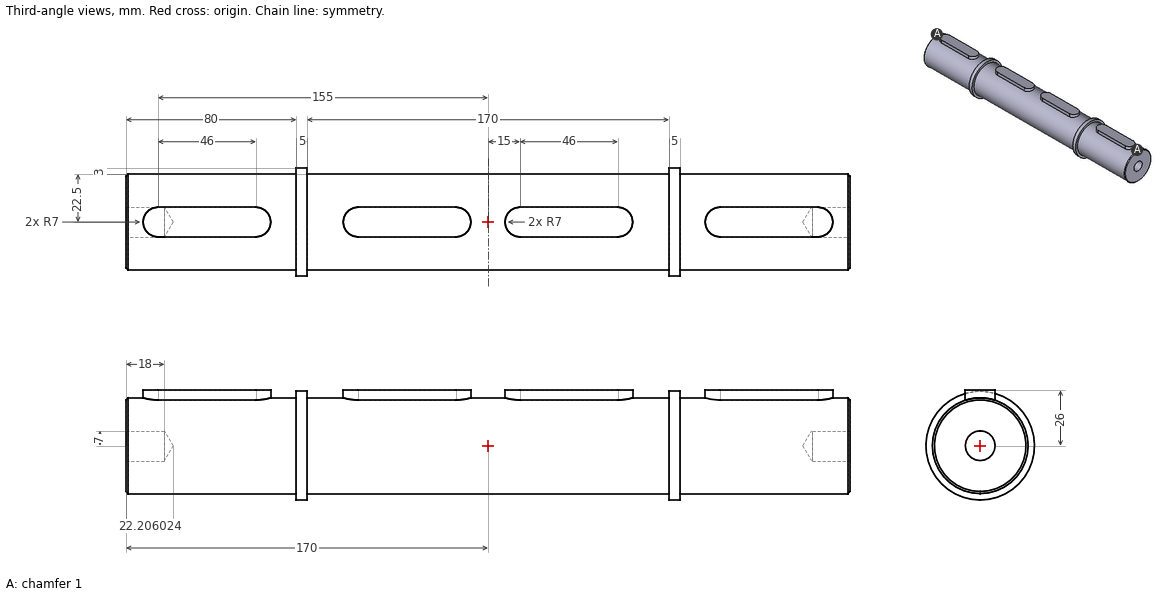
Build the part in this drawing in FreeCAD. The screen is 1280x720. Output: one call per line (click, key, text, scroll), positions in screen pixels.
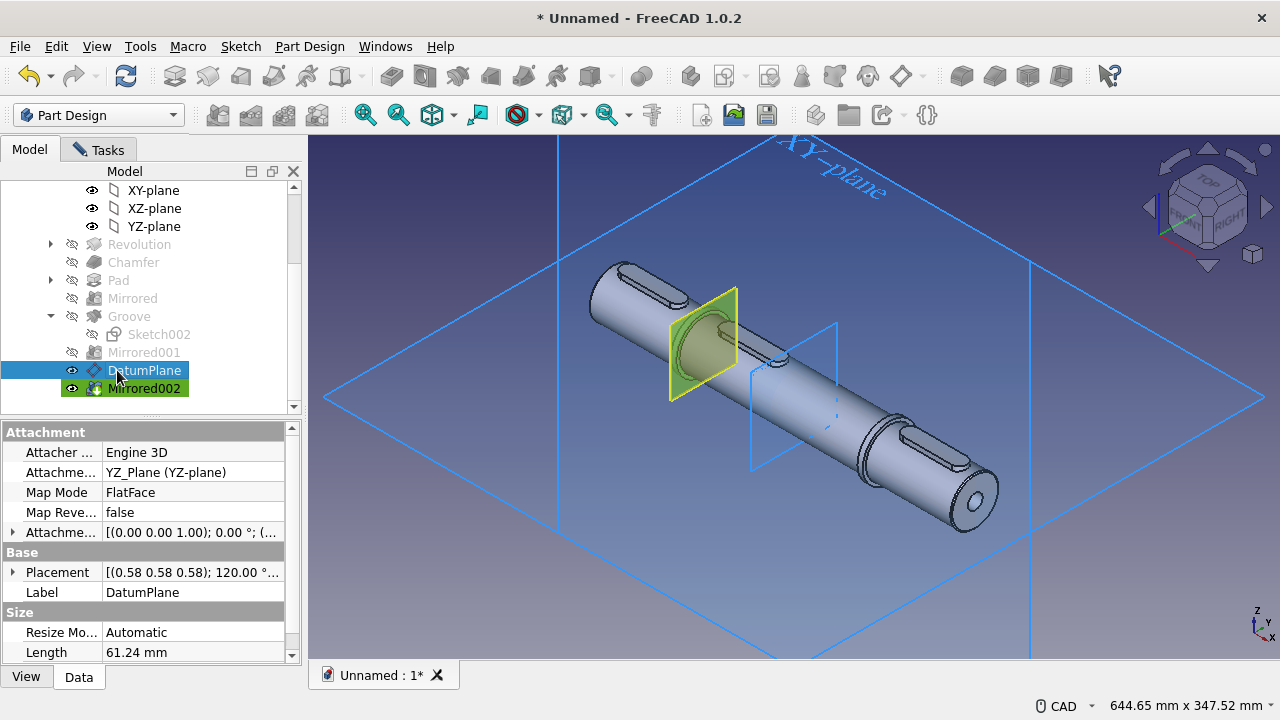
click(98, 149)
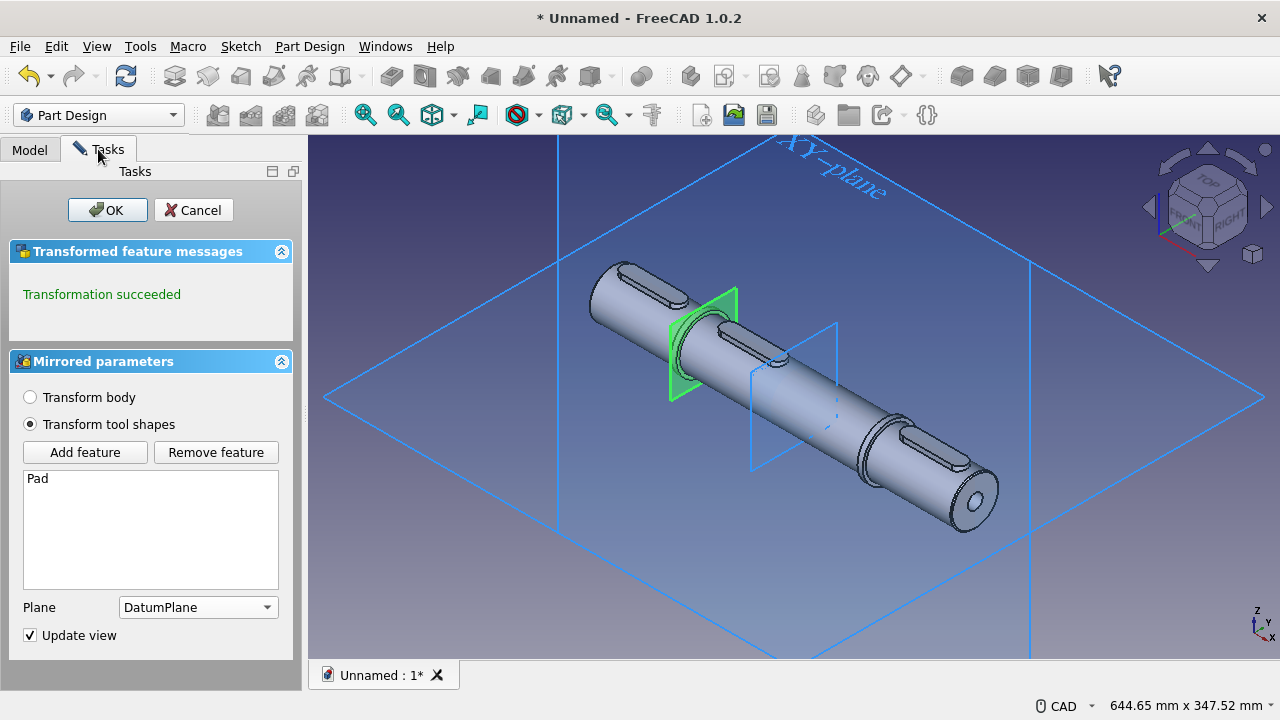
click(108, 210)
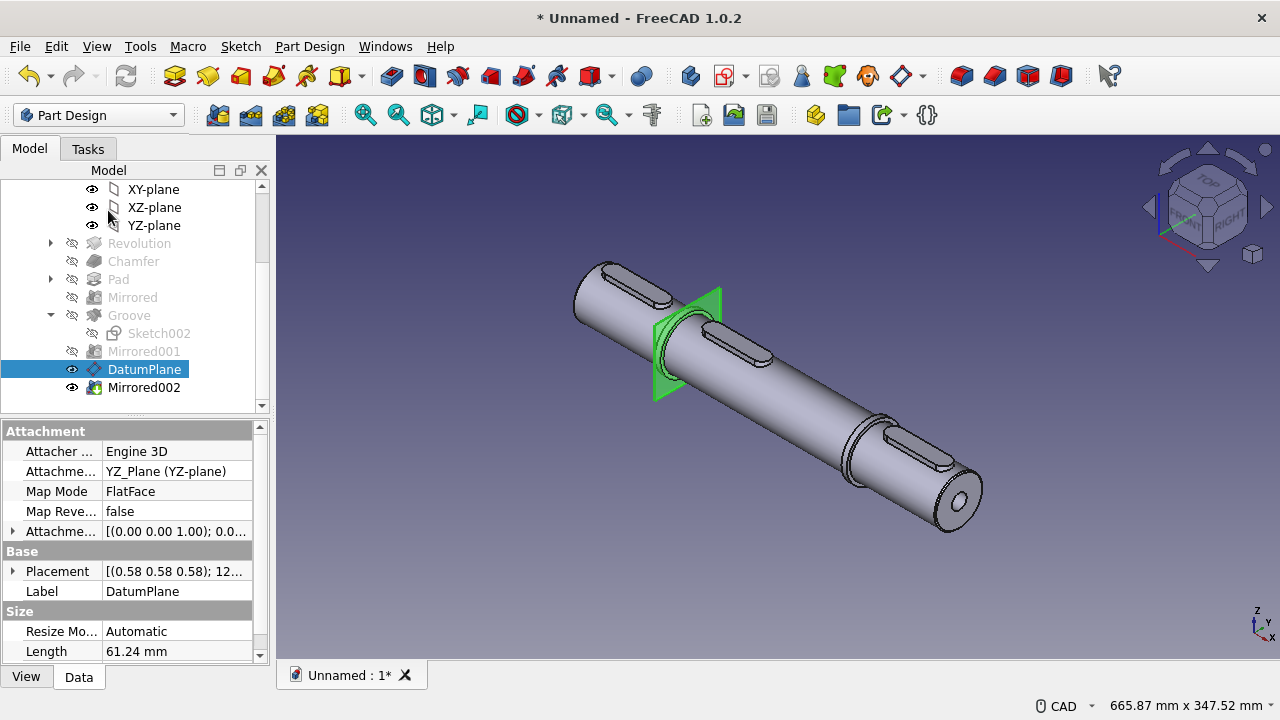
click(117, 369)
key(space)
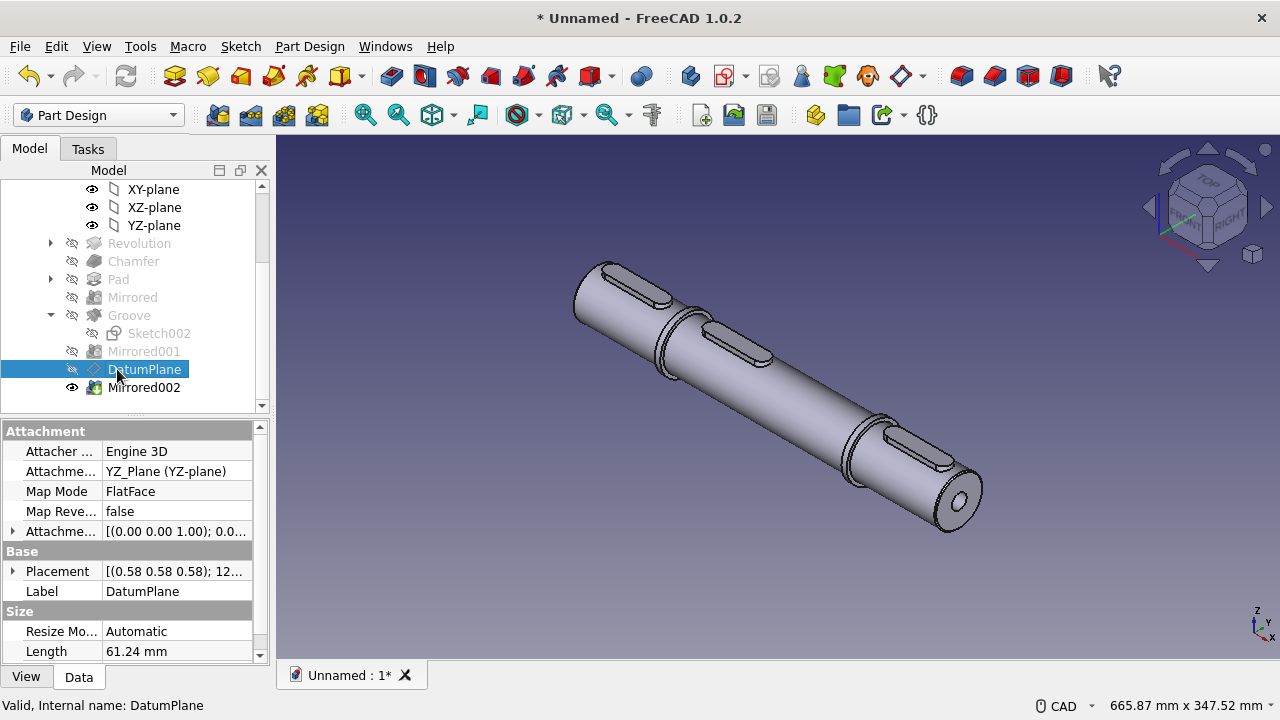
click(316, 619)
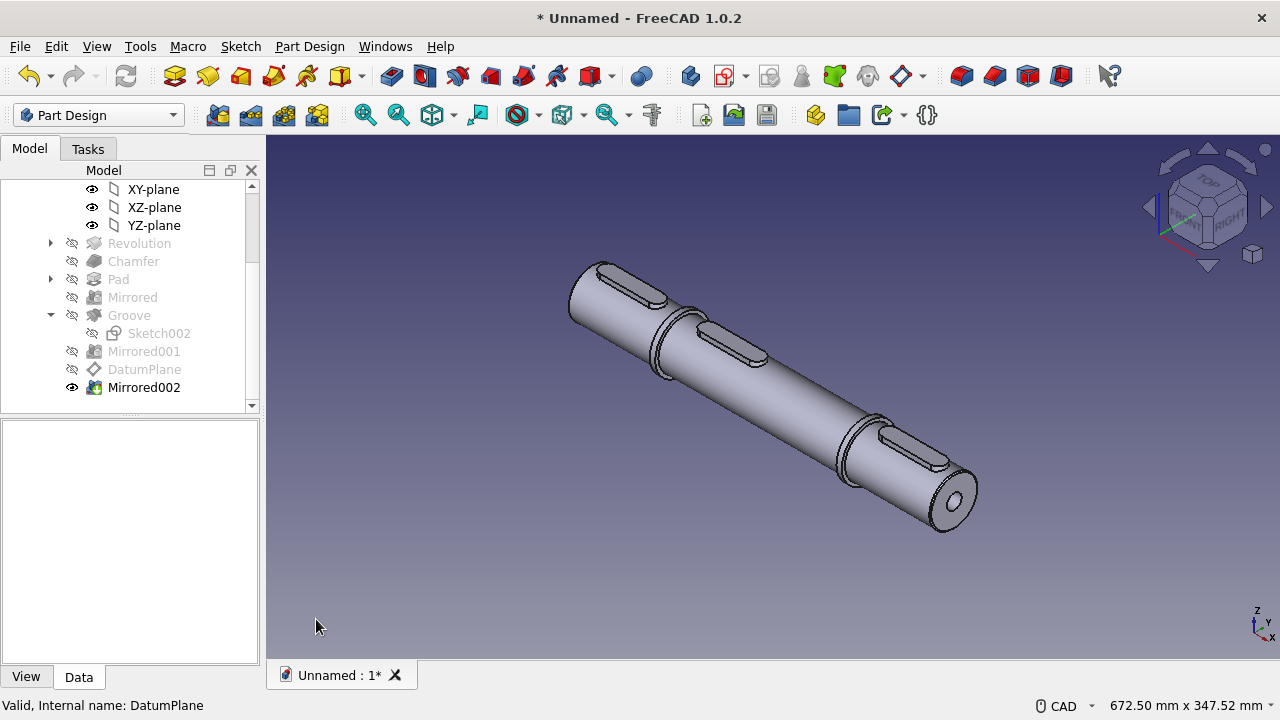
click(724, 76)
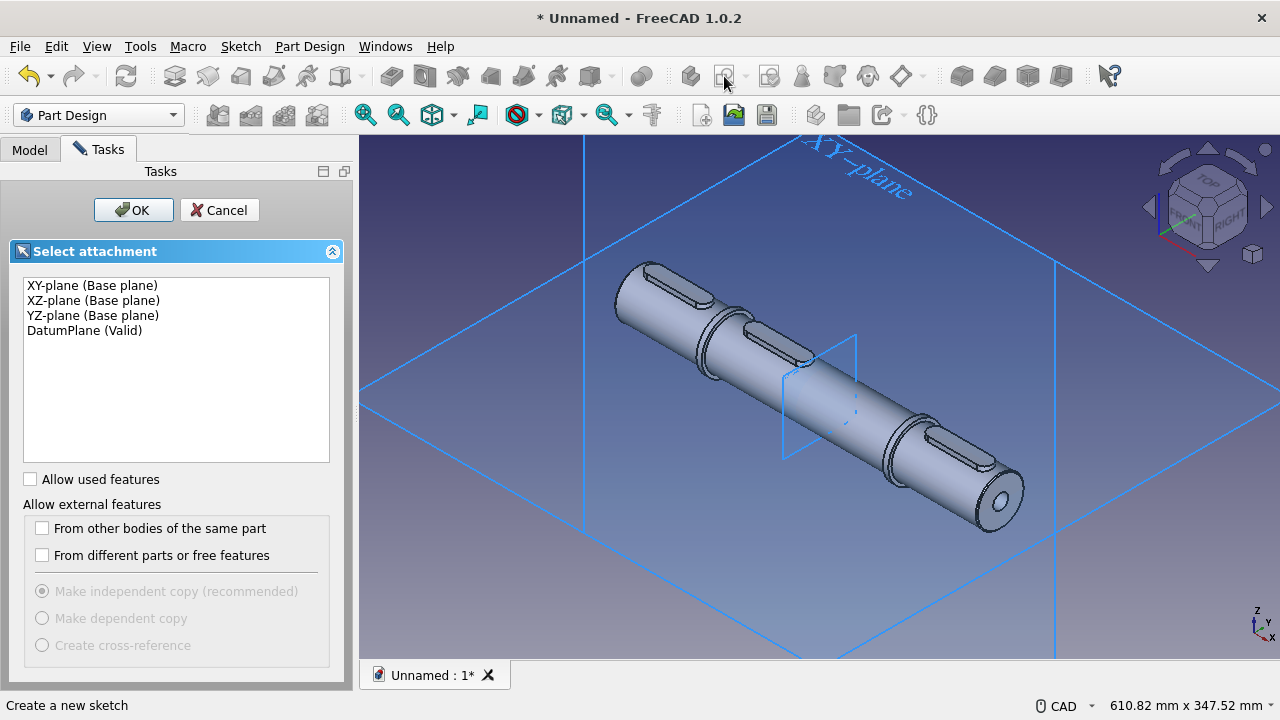
click(84, 286)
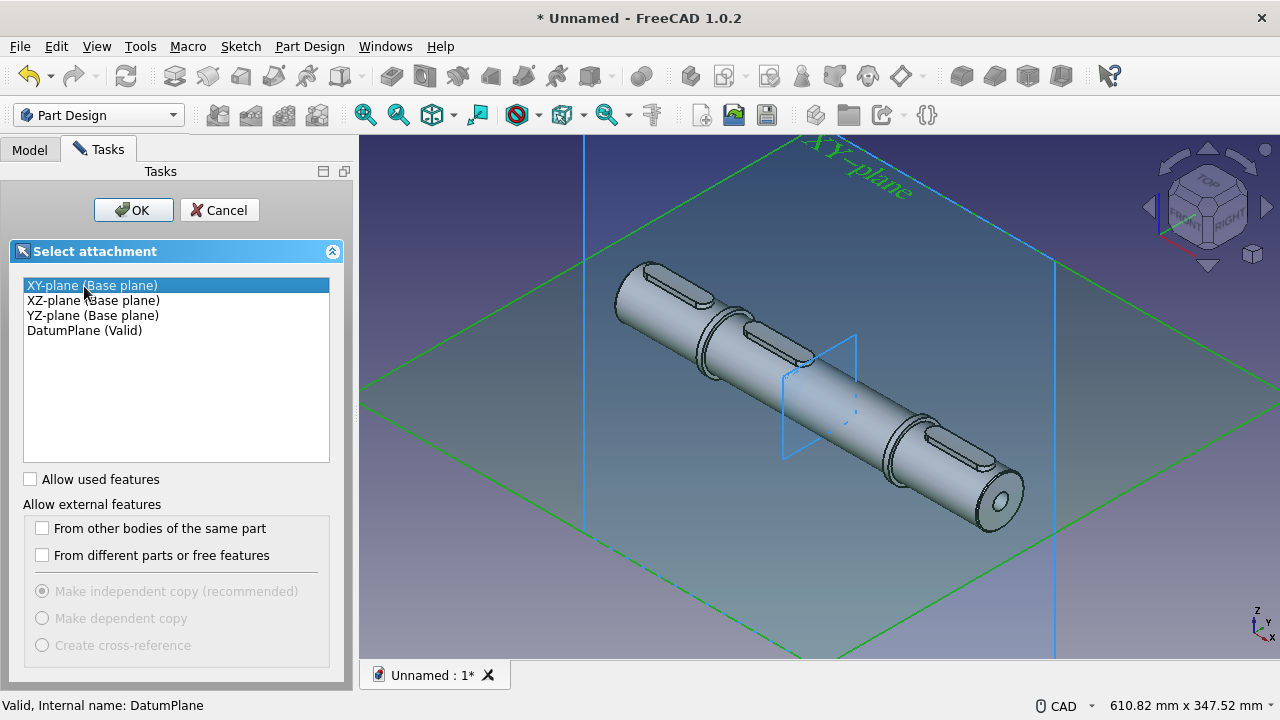
click(134, 210)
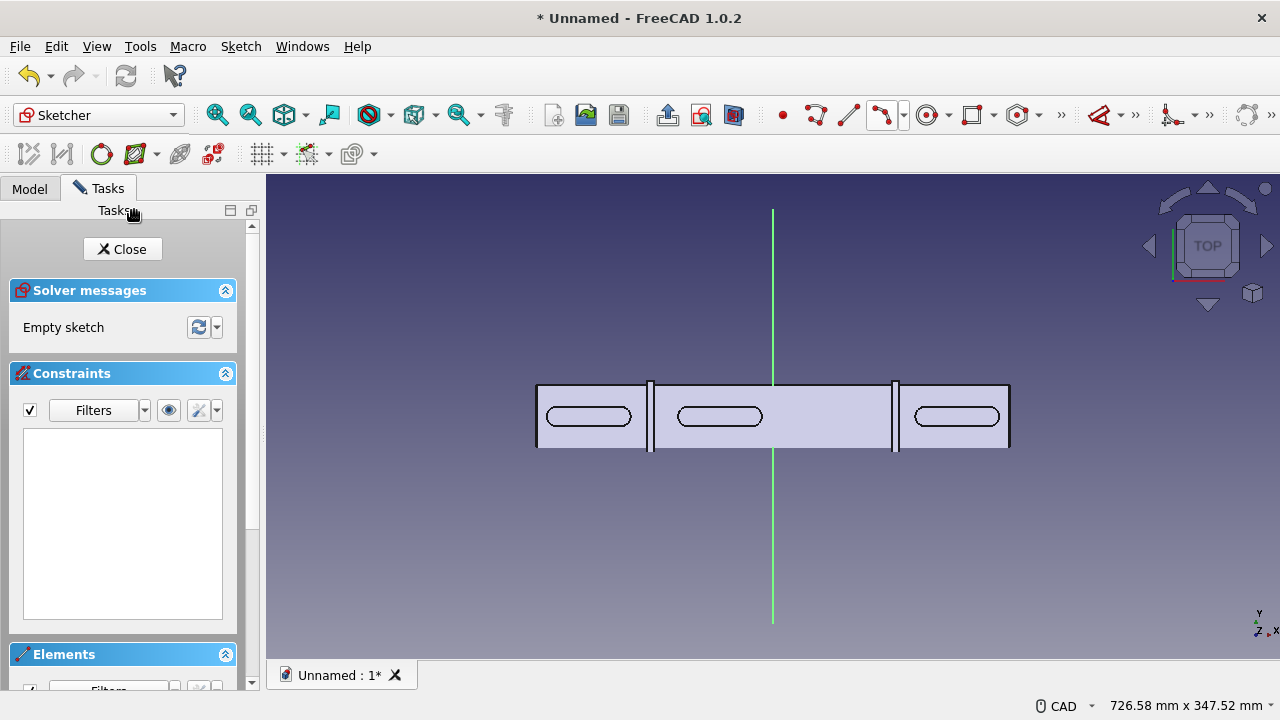
click(734, 116)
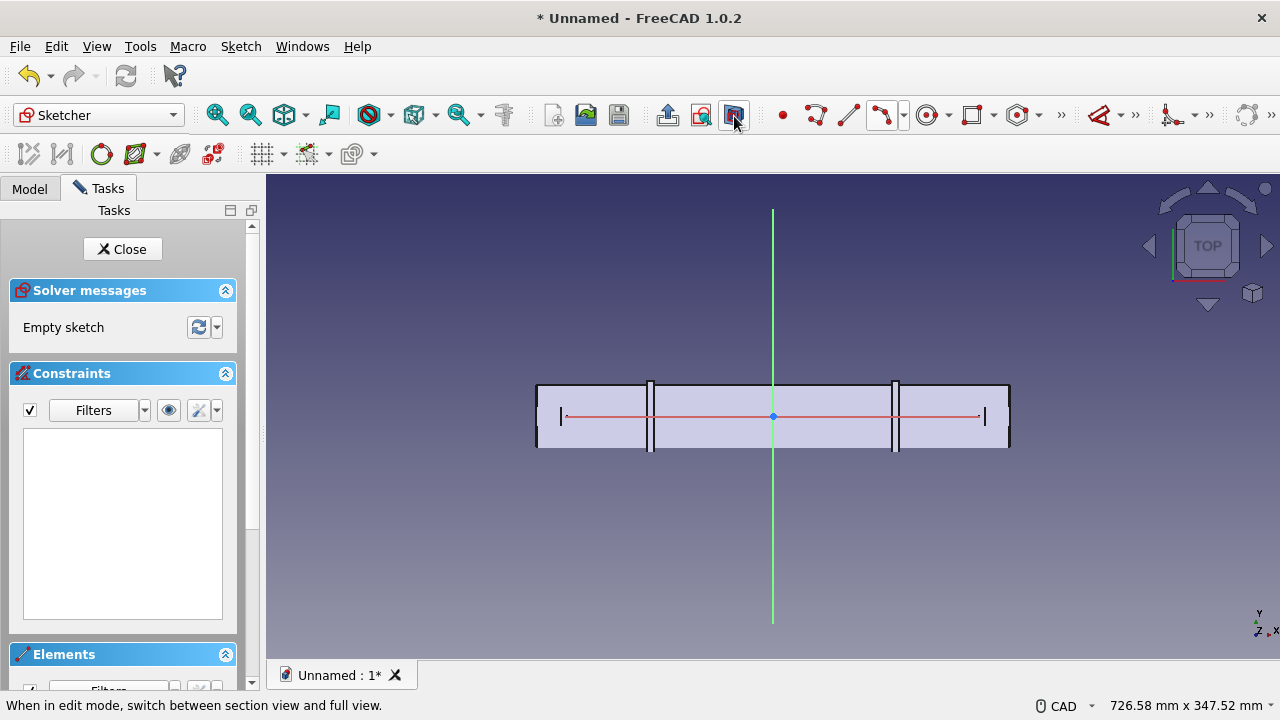
scroll(843, 416, up, 9)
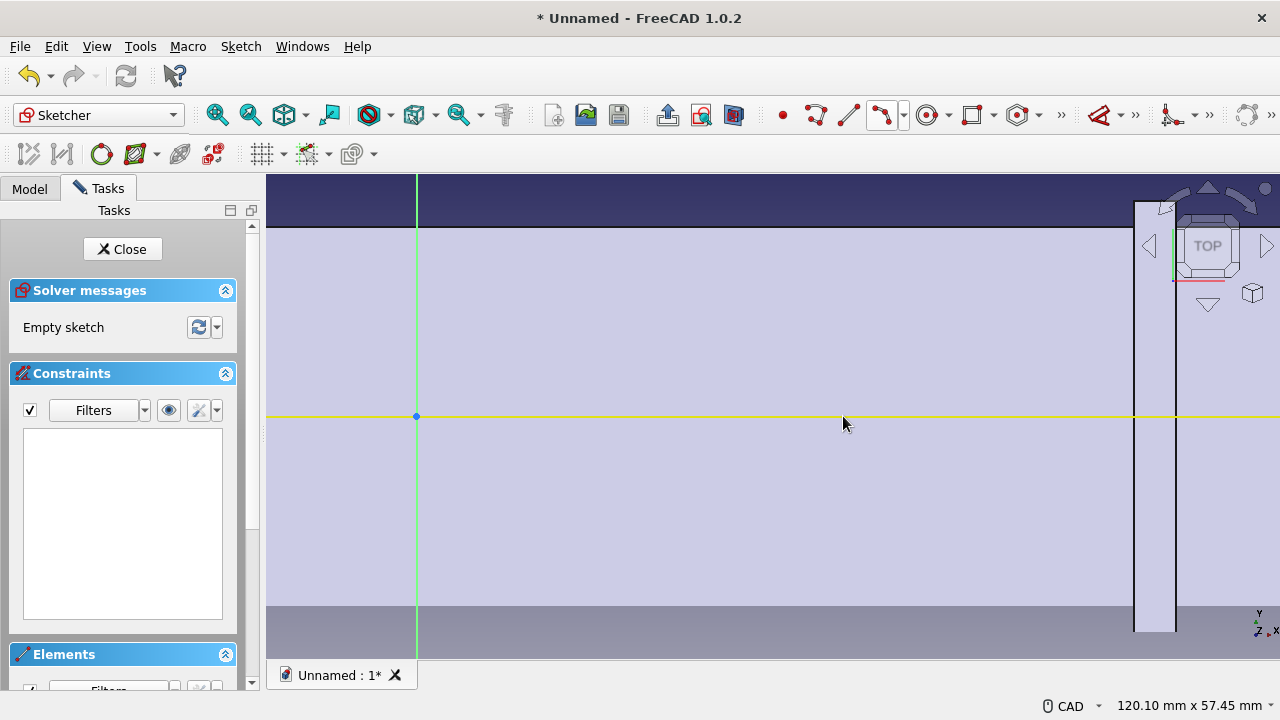
key(g)
key(s)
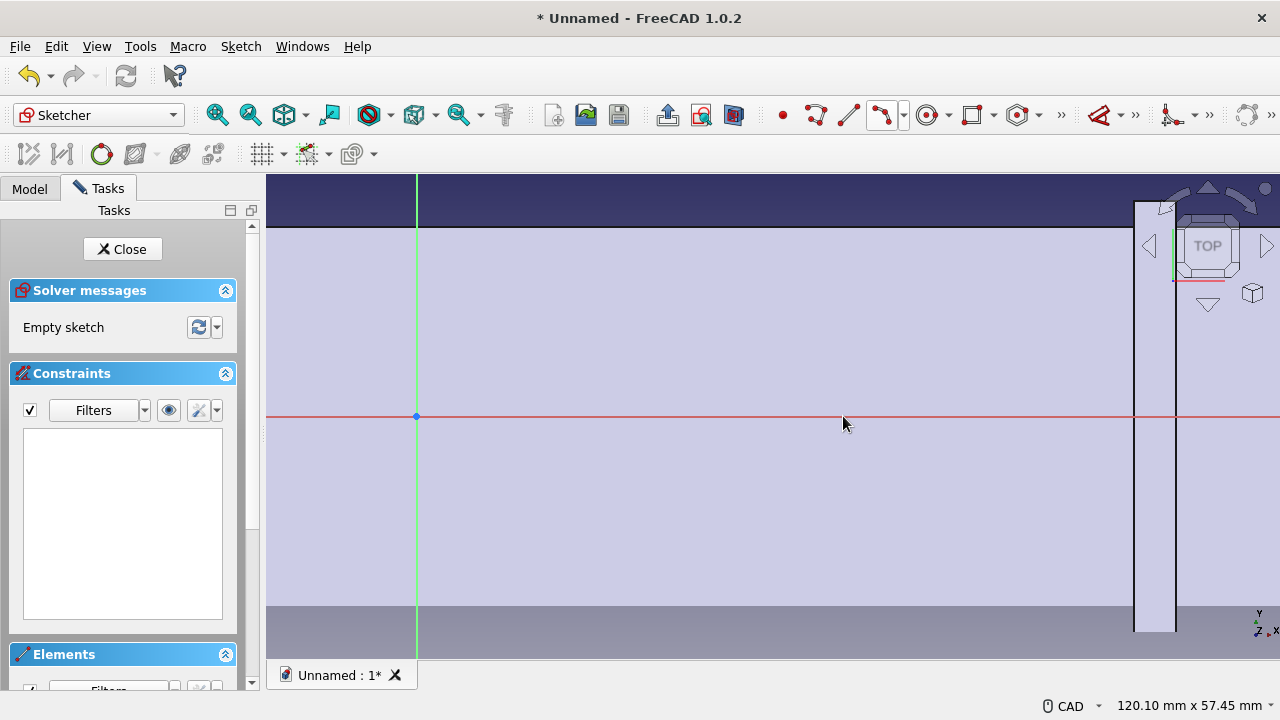
click(543, 416)